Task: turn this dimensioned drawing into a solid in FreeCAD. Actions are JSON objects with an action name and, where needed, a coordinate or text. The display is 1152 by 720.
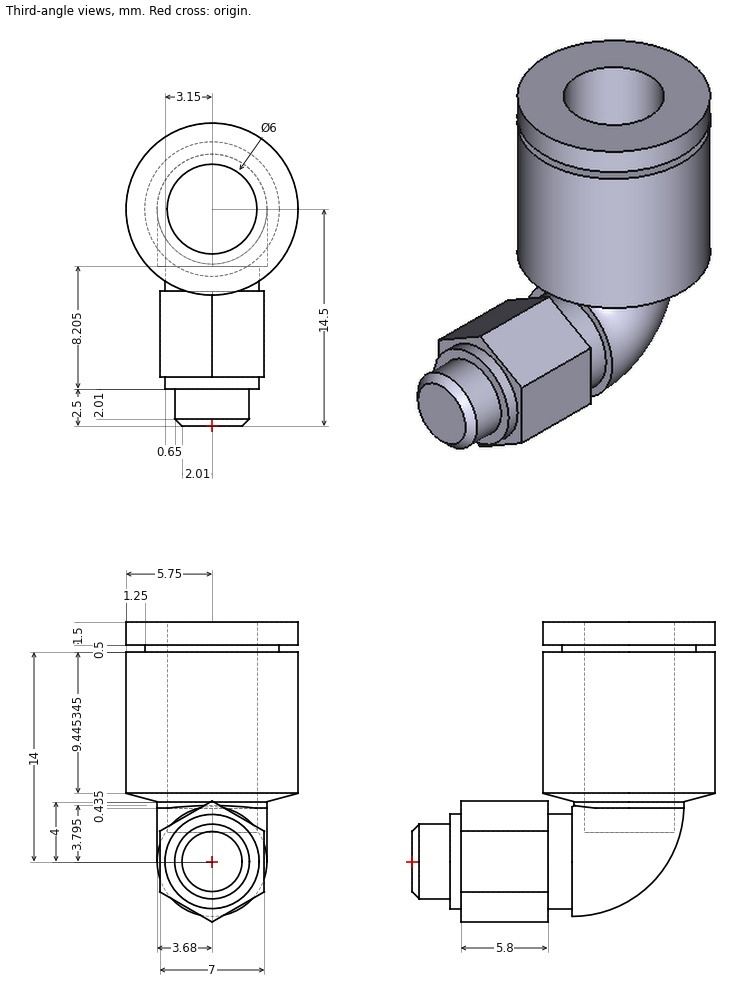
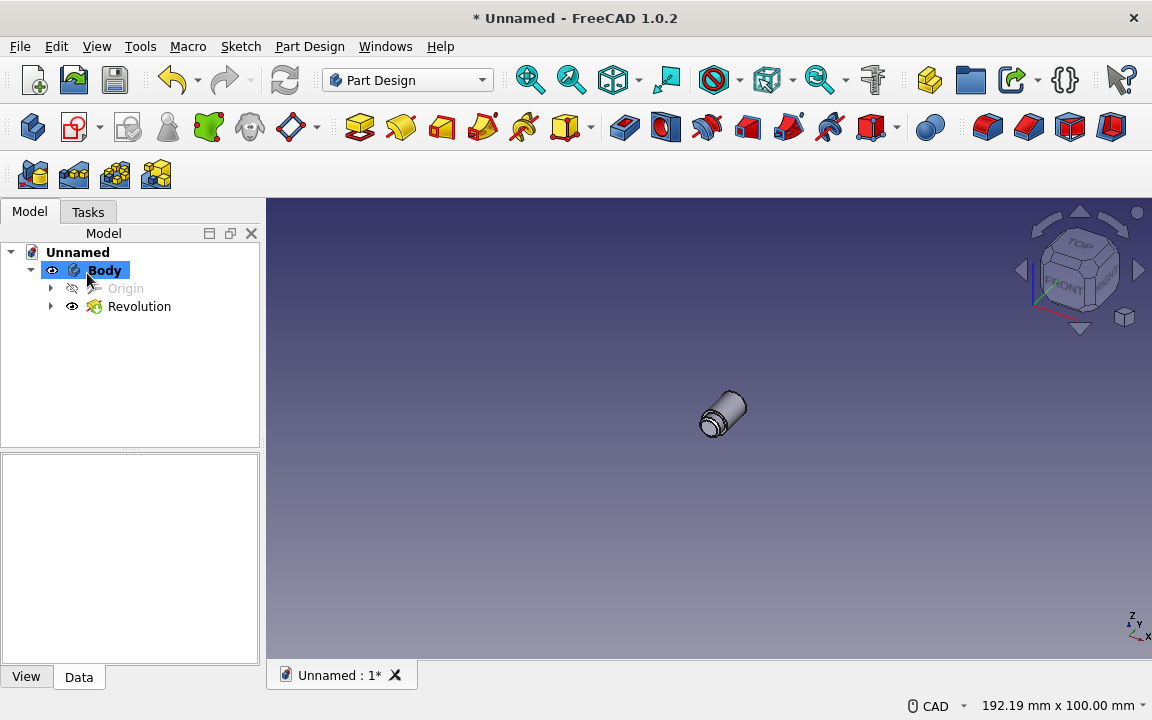
{"action": "left_click", "coordinate": [531, 80]}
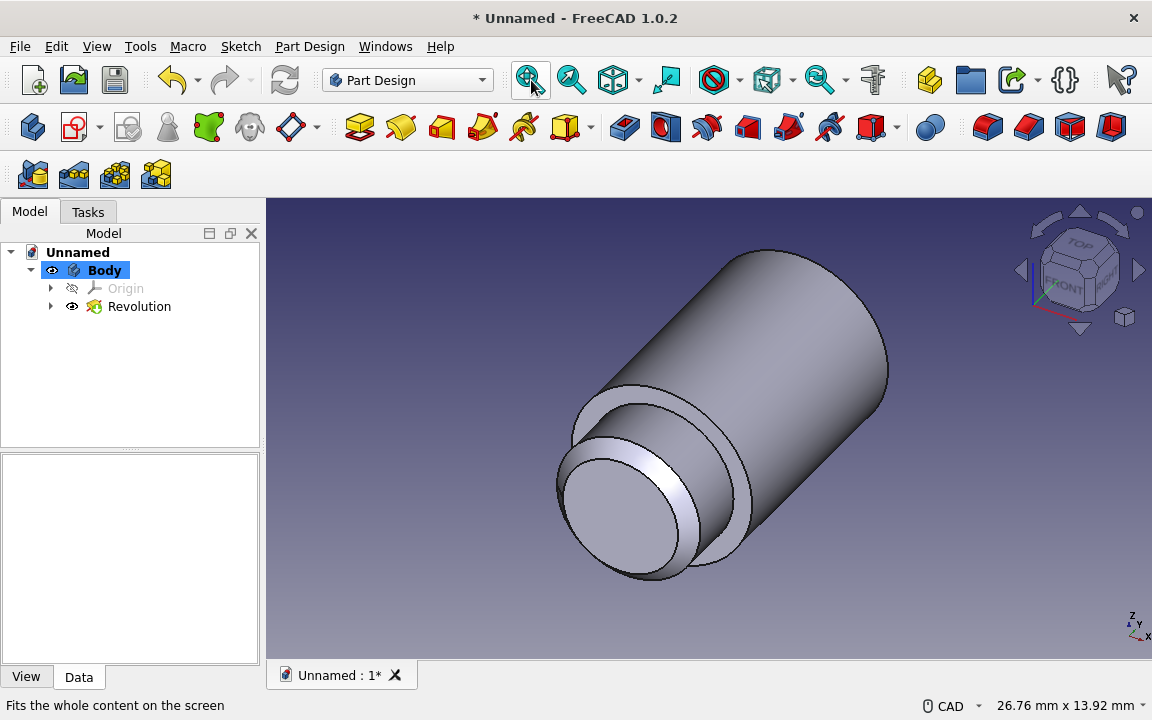
{"action": "key", "text": "4"}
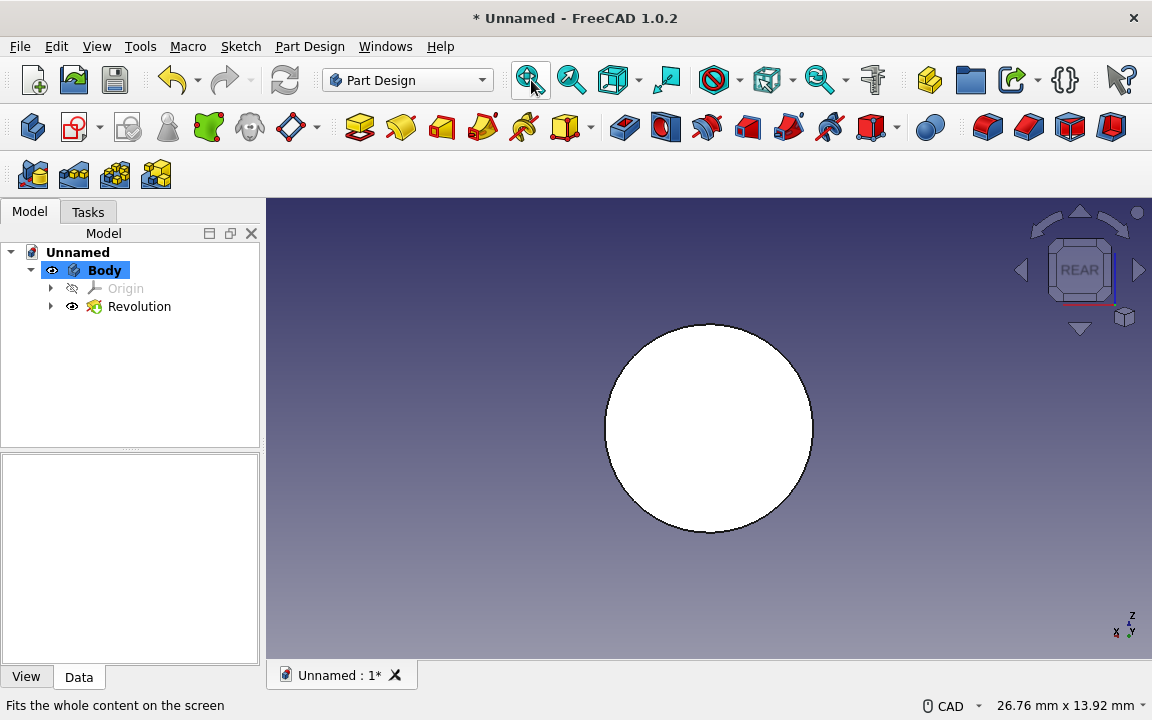
{"action": "left_click", "coordinate": [709, 427]}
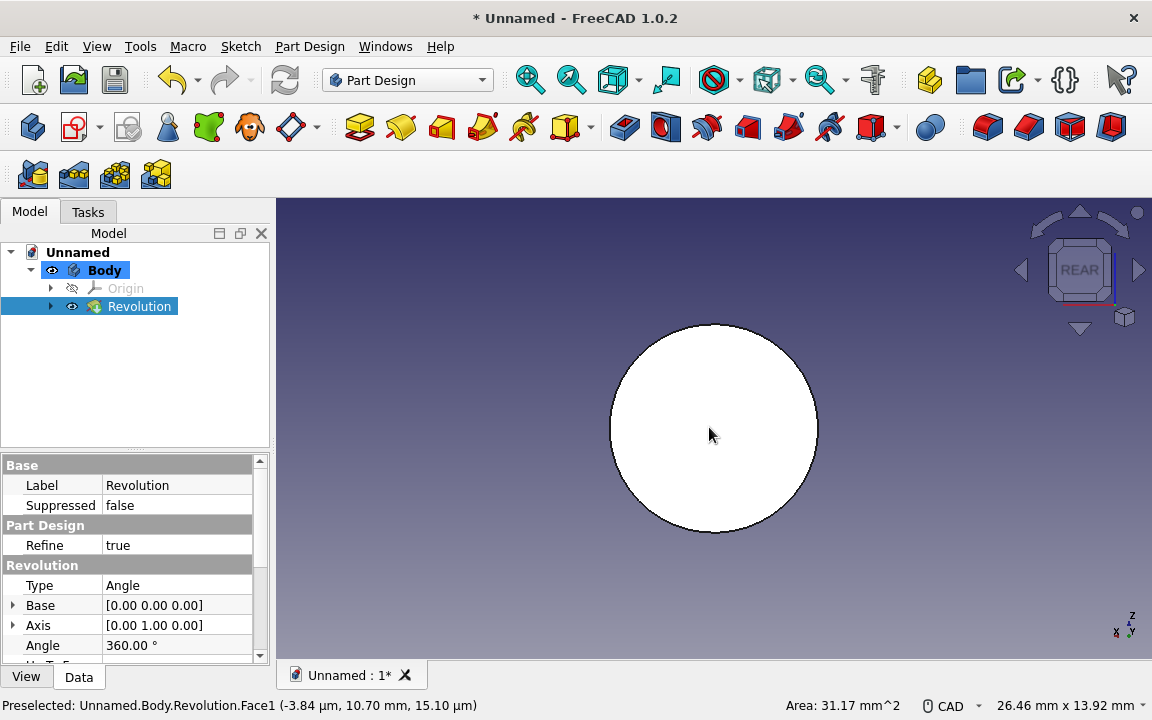
{"action": "left_click", "coordinate": [74, 128]}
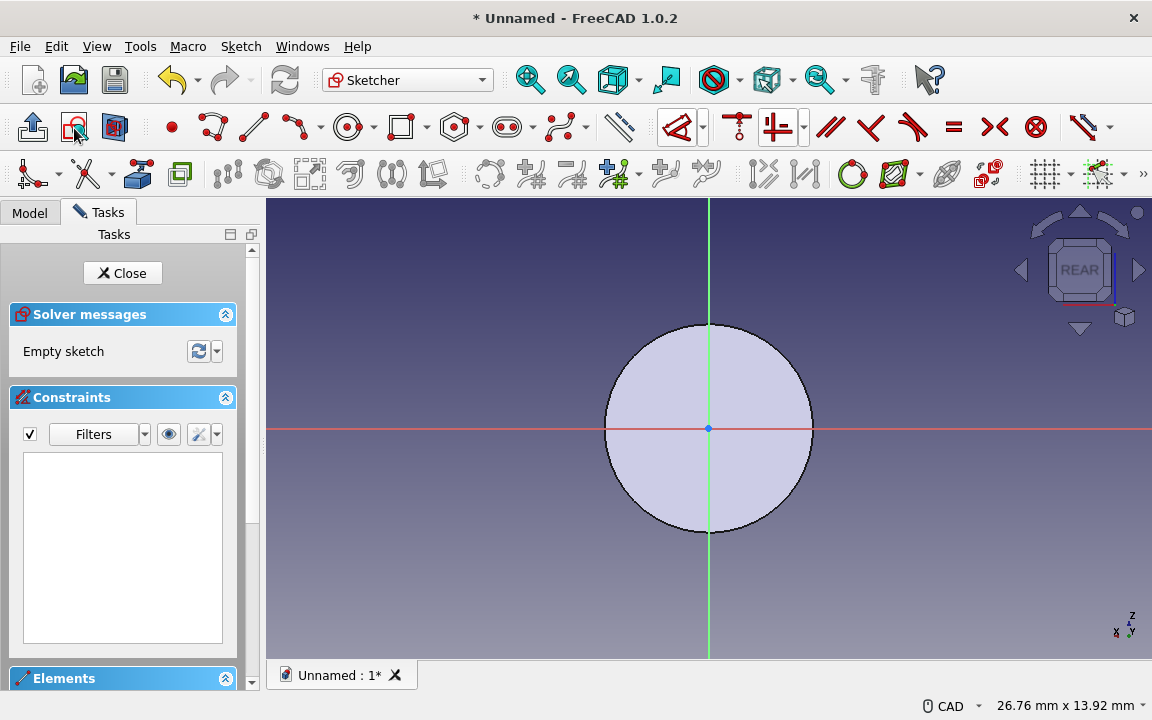
{"action": "left_click", "coordinate": [348, 128]}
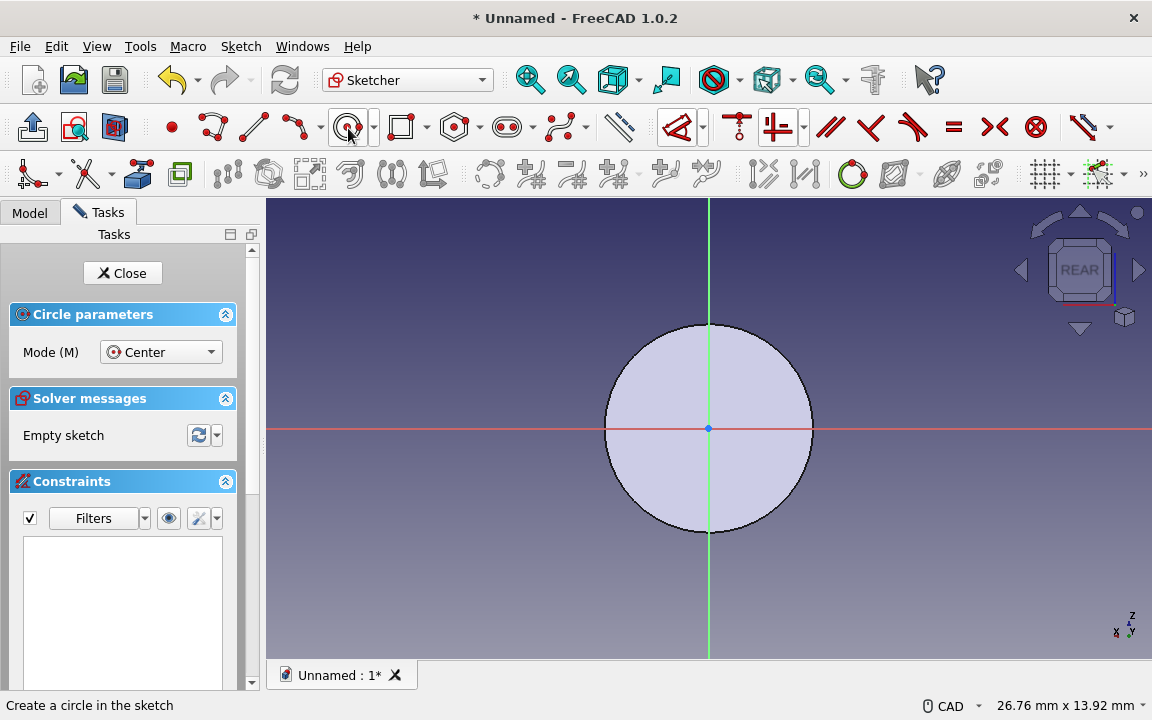
{"action": "left_click", "coordinate": [709, 428]}
{"action": "left_click", "coordinate": [795, 343]}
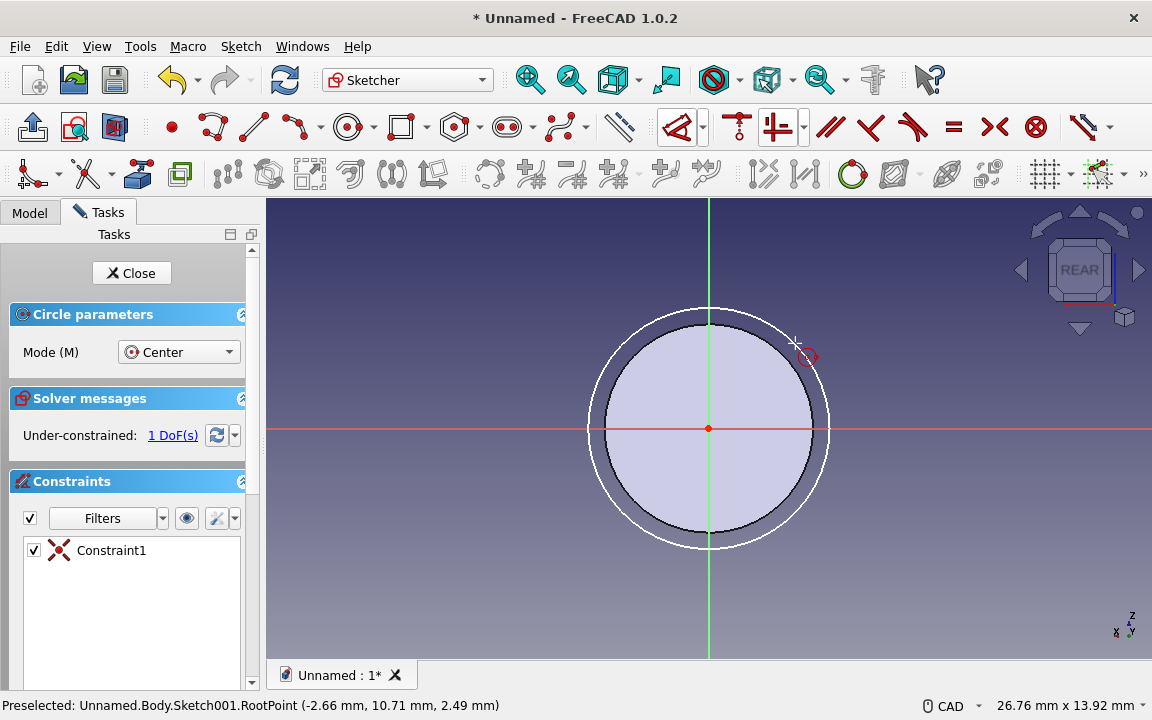
{"action": "left_click", "coordinate": [254, 128]}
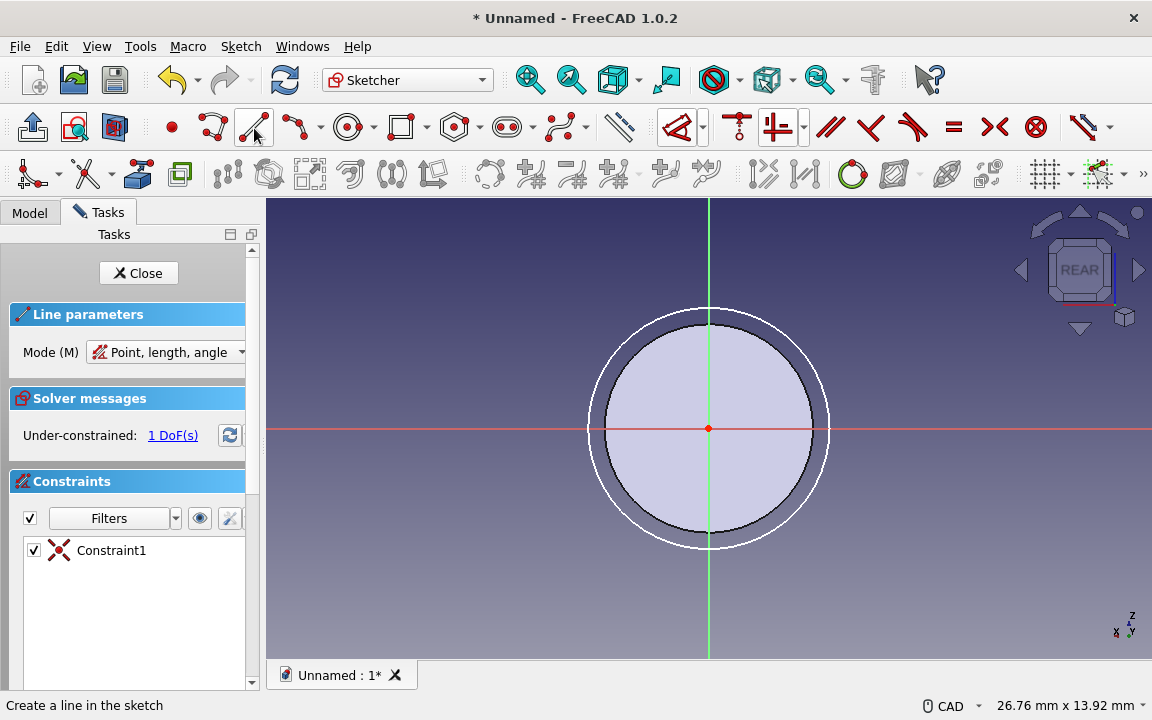
{"action": "left_click", "coordinate": [855, 303]}
{"action": "left_click", "coordinate": [563, 303]}
{"action": "key", "text": "Escape"}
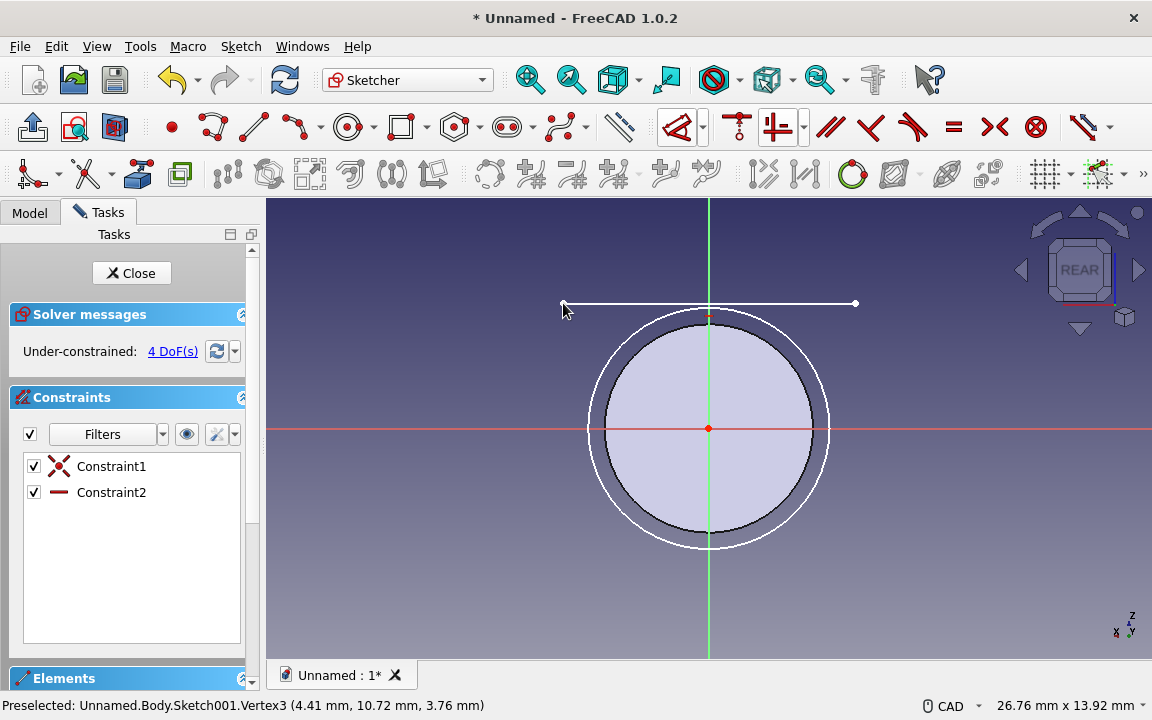
{"action": "left_click", "coordinate": [767, 304]}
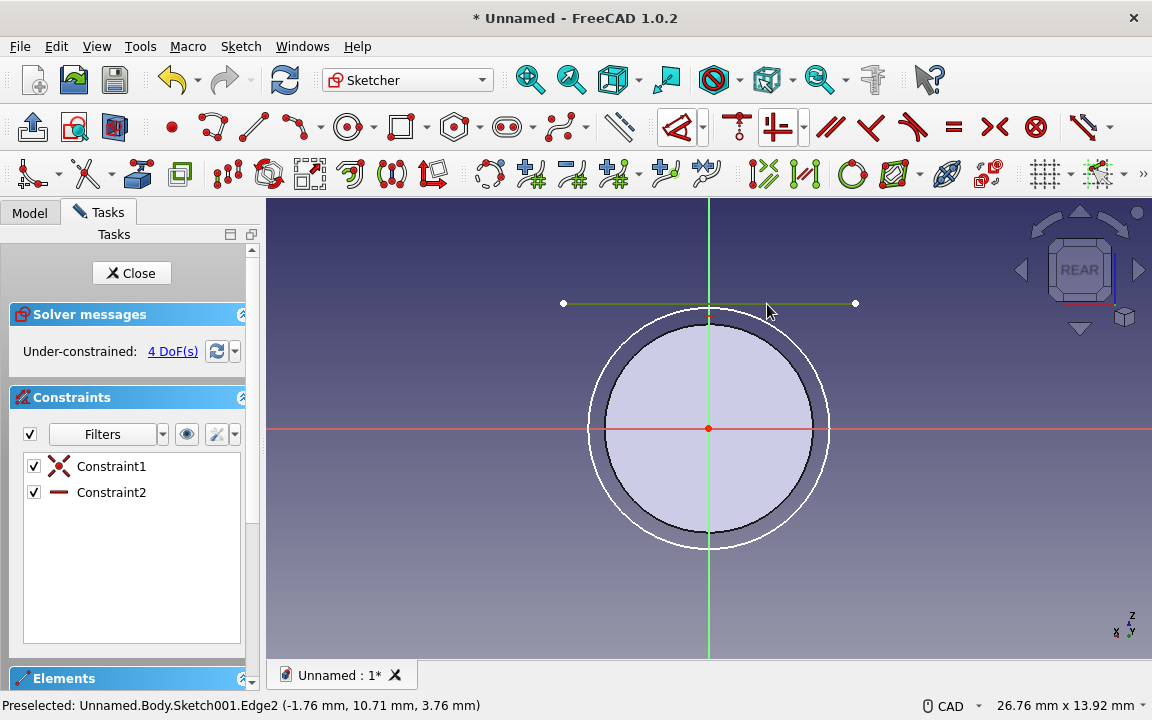
{"action": "left_click", "coordinate": [620, 128]}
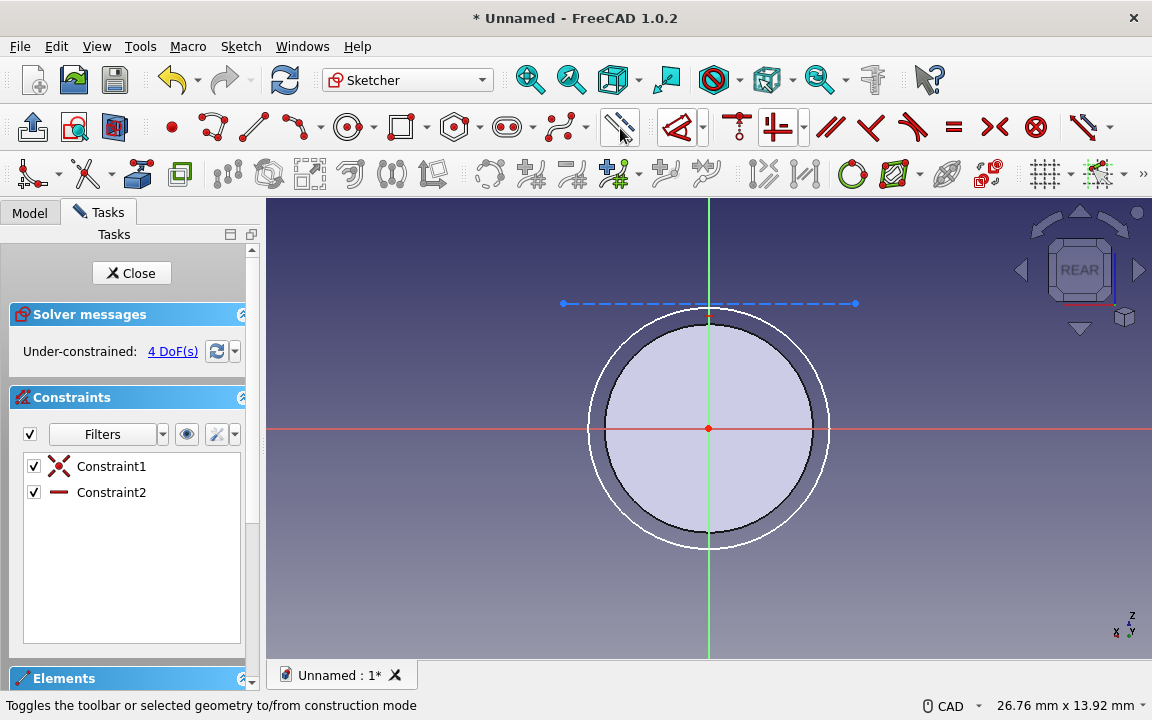
{"action": "left_click", "coordinate": [794, 343]}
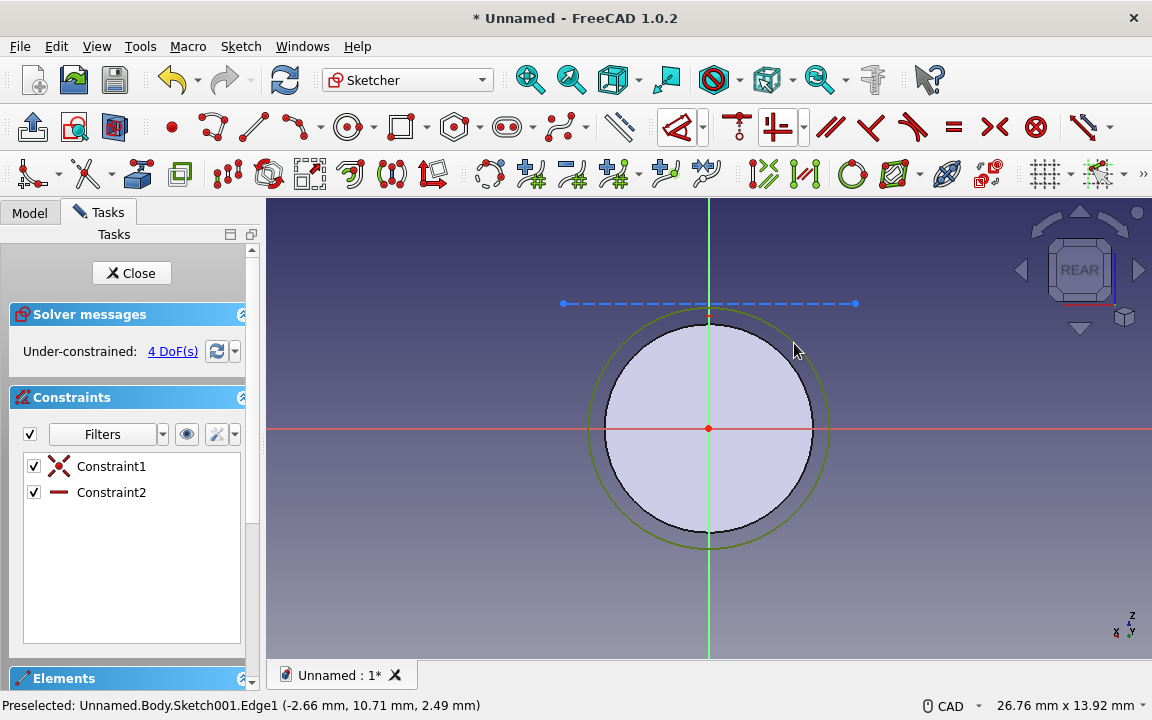
{"action": "left_click", "coordinate": [702, 128]}